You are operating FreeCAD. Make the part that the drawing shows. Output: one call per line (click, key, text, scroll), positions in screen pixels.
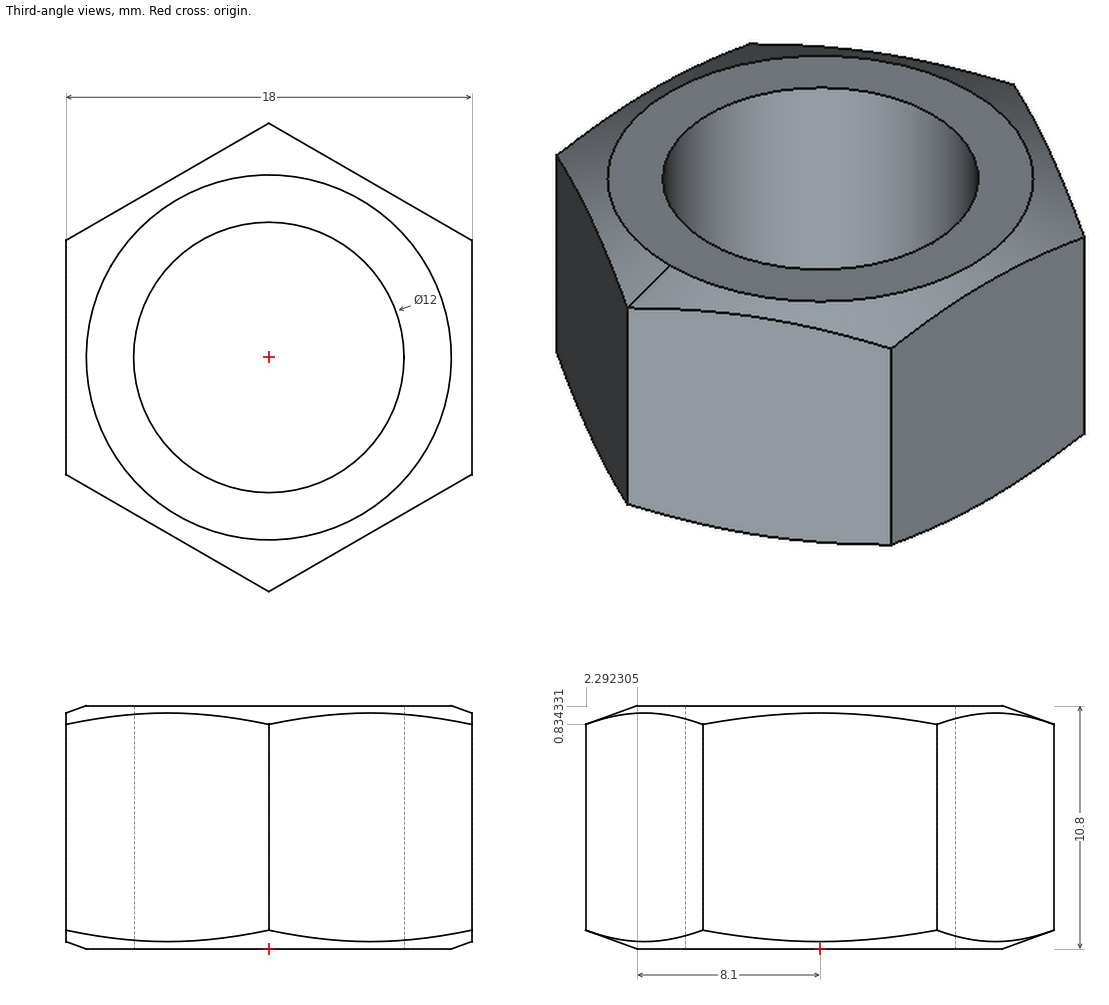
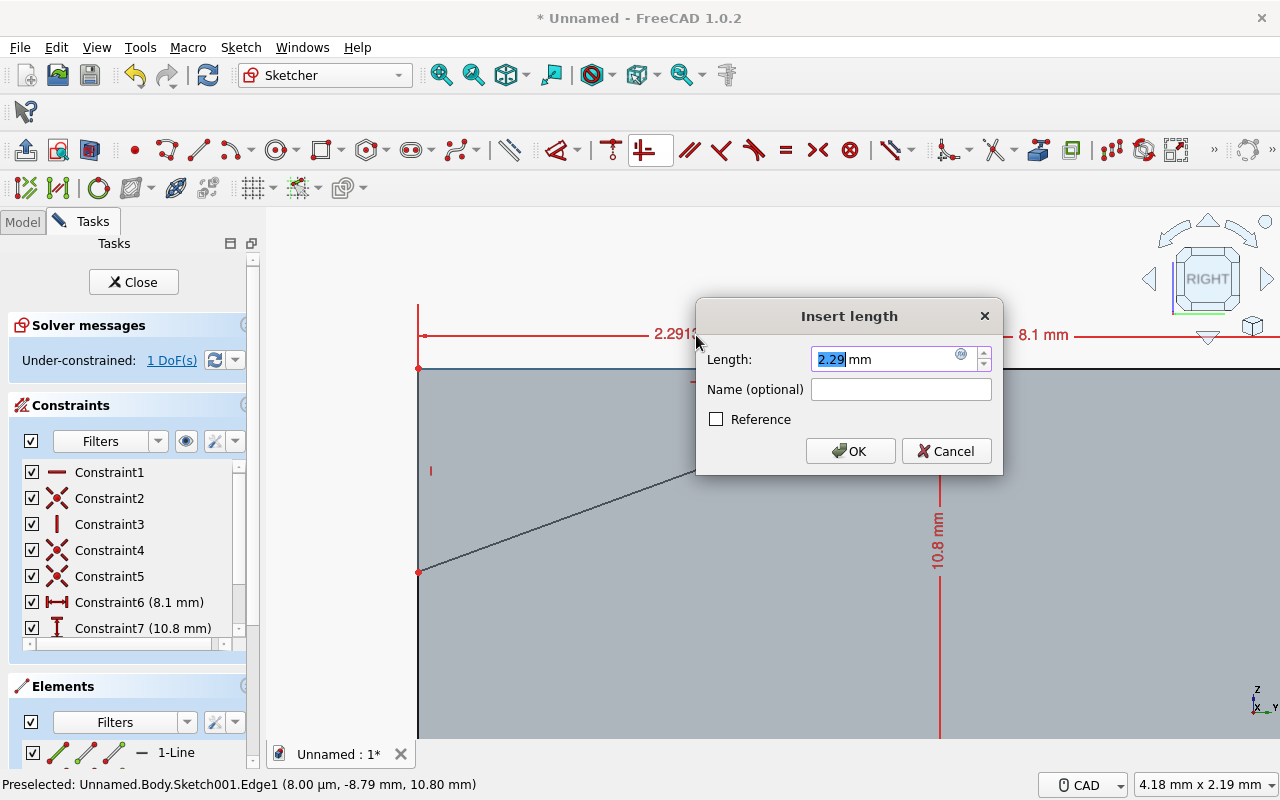
text(2.292305)
key(Return)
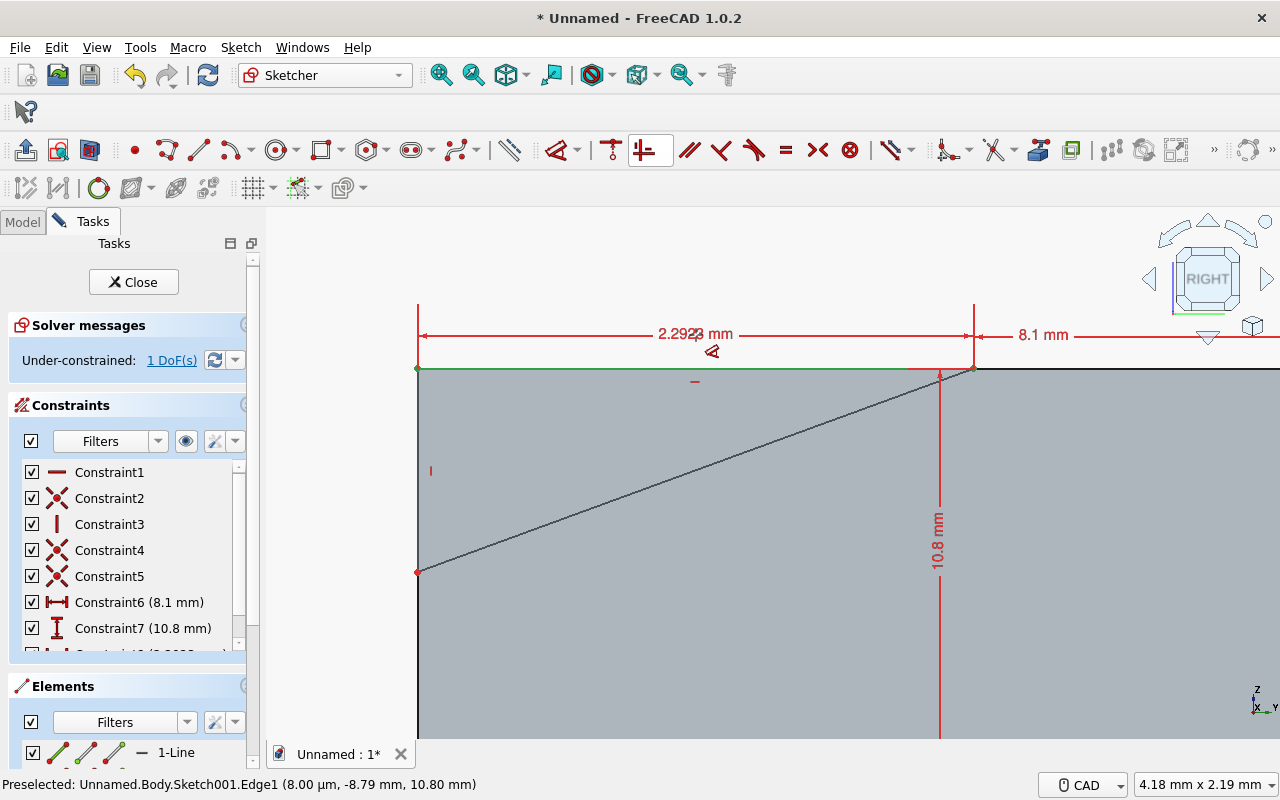
click(418, 430)
click(384, 470)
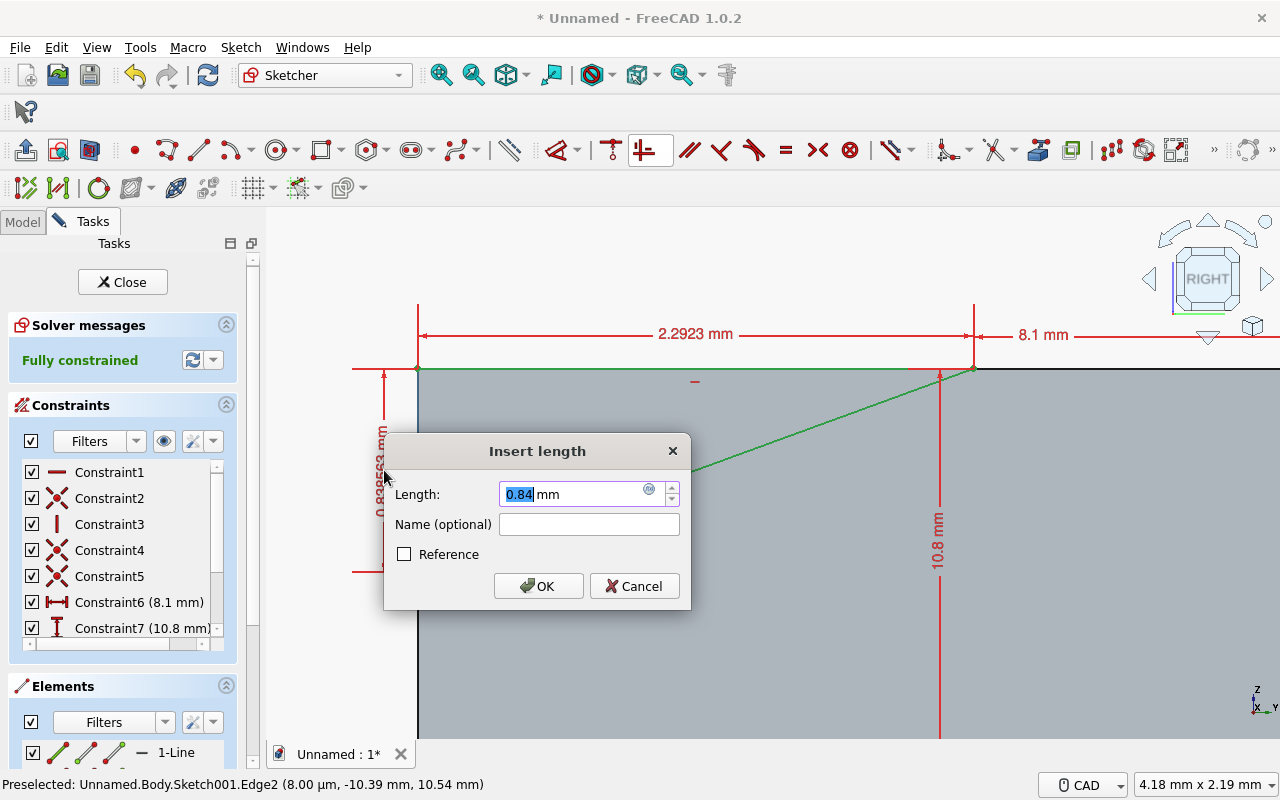
text(0.834331)
key(Return)
key(Escape)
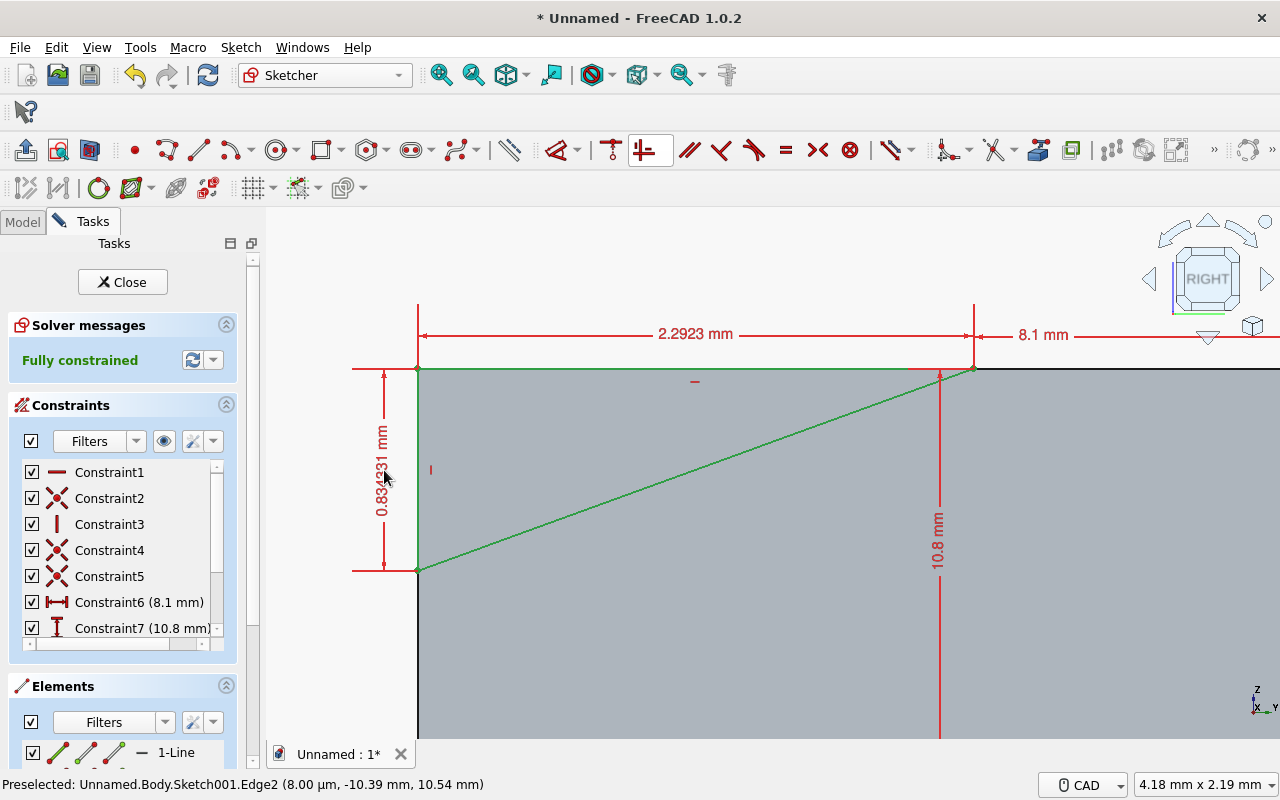
click(123, 282)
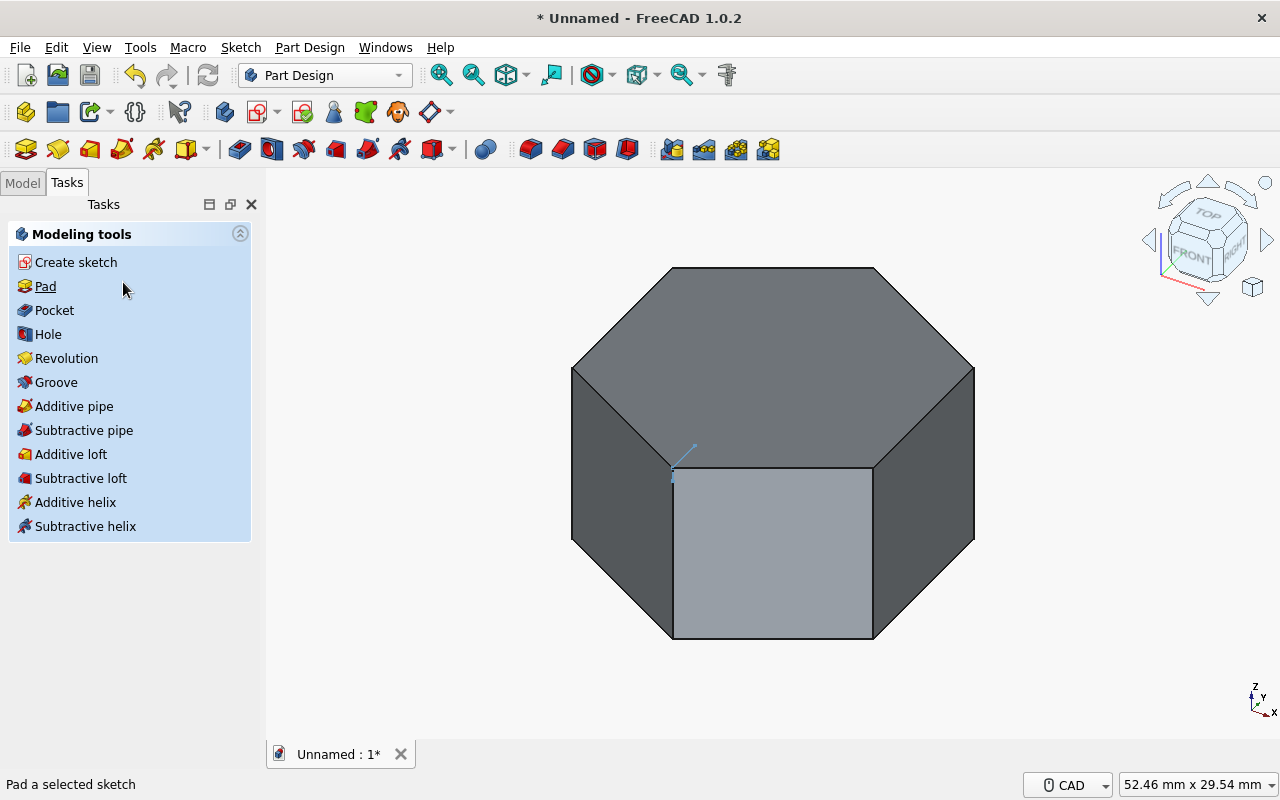
click(304, 150)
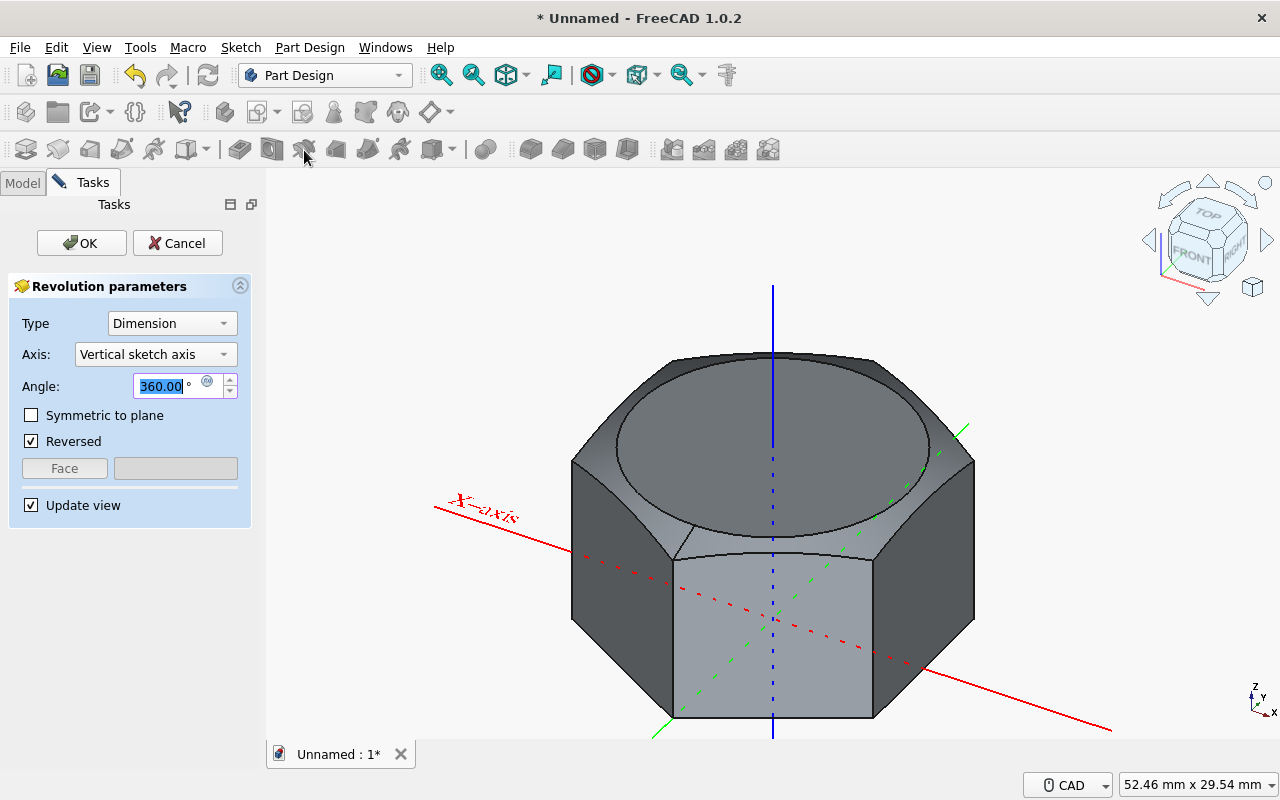
click(82, 243)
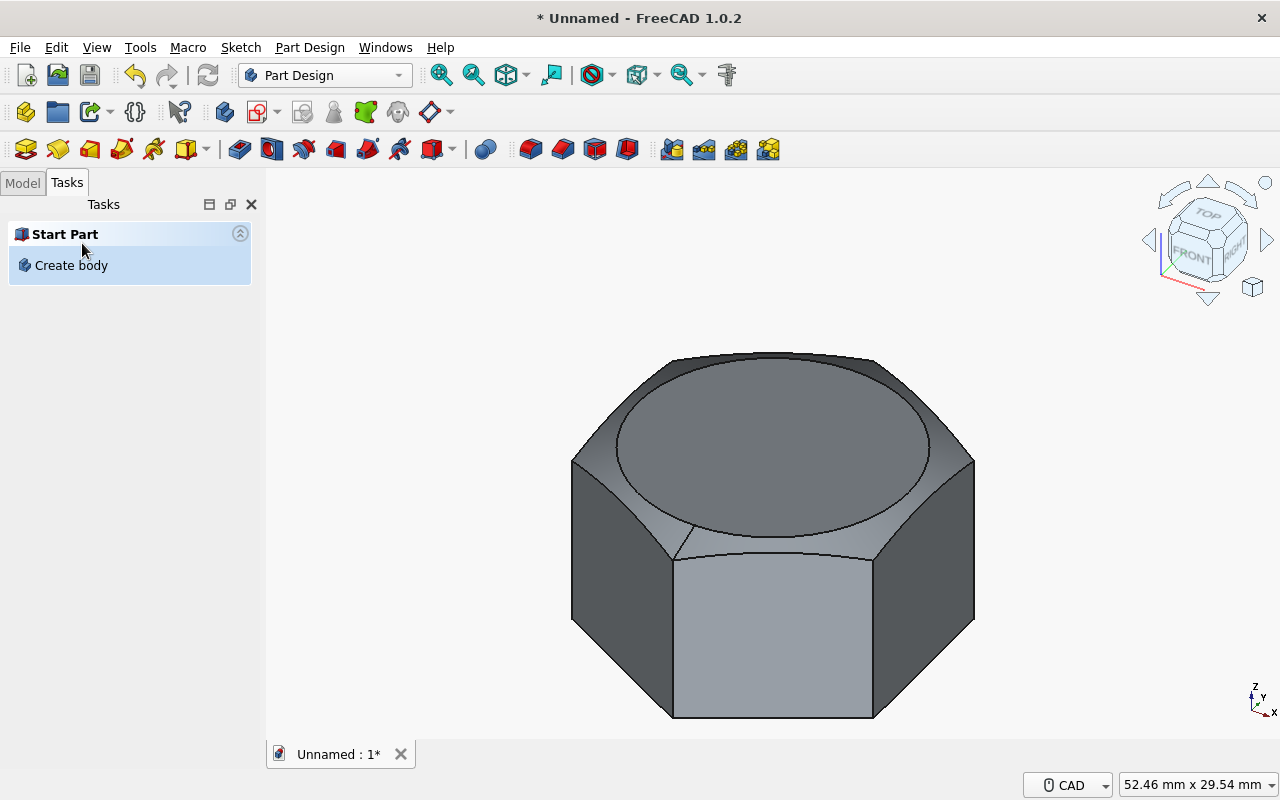
click(442, 76)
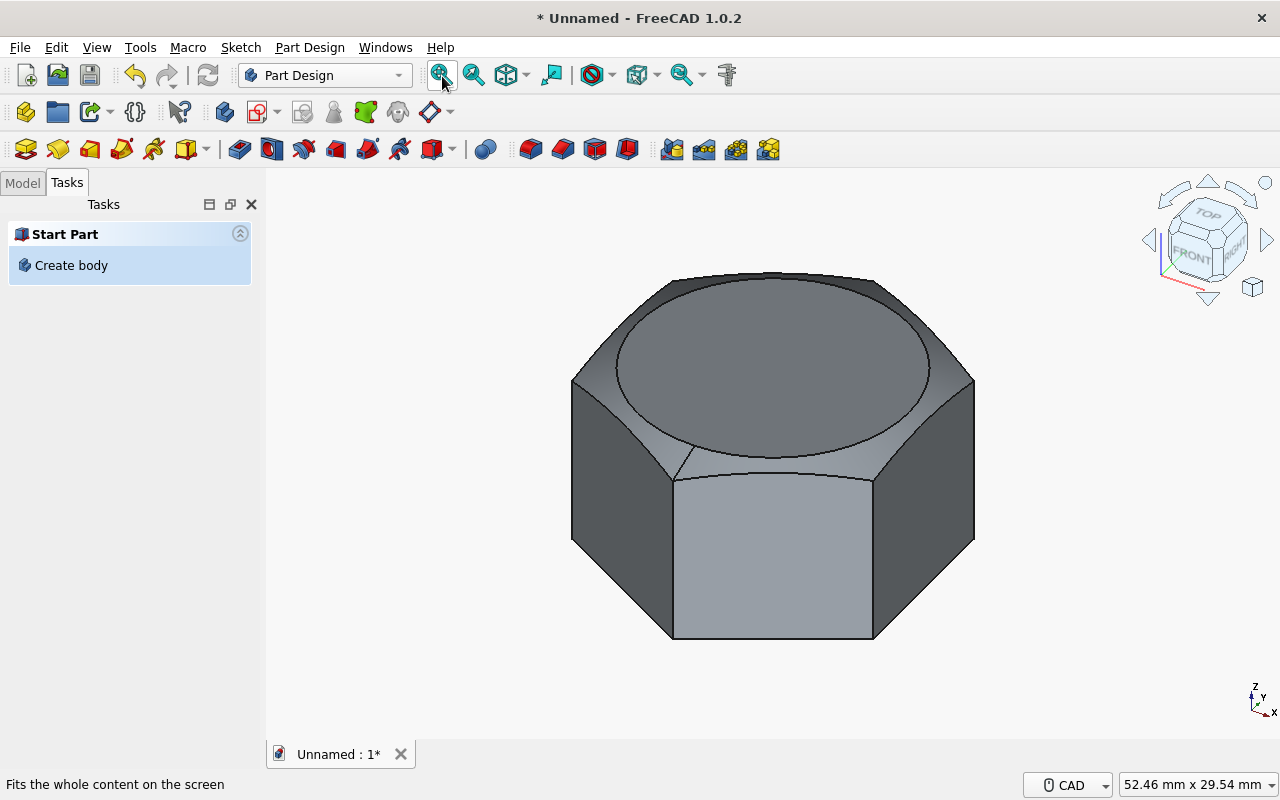
click(23, 182)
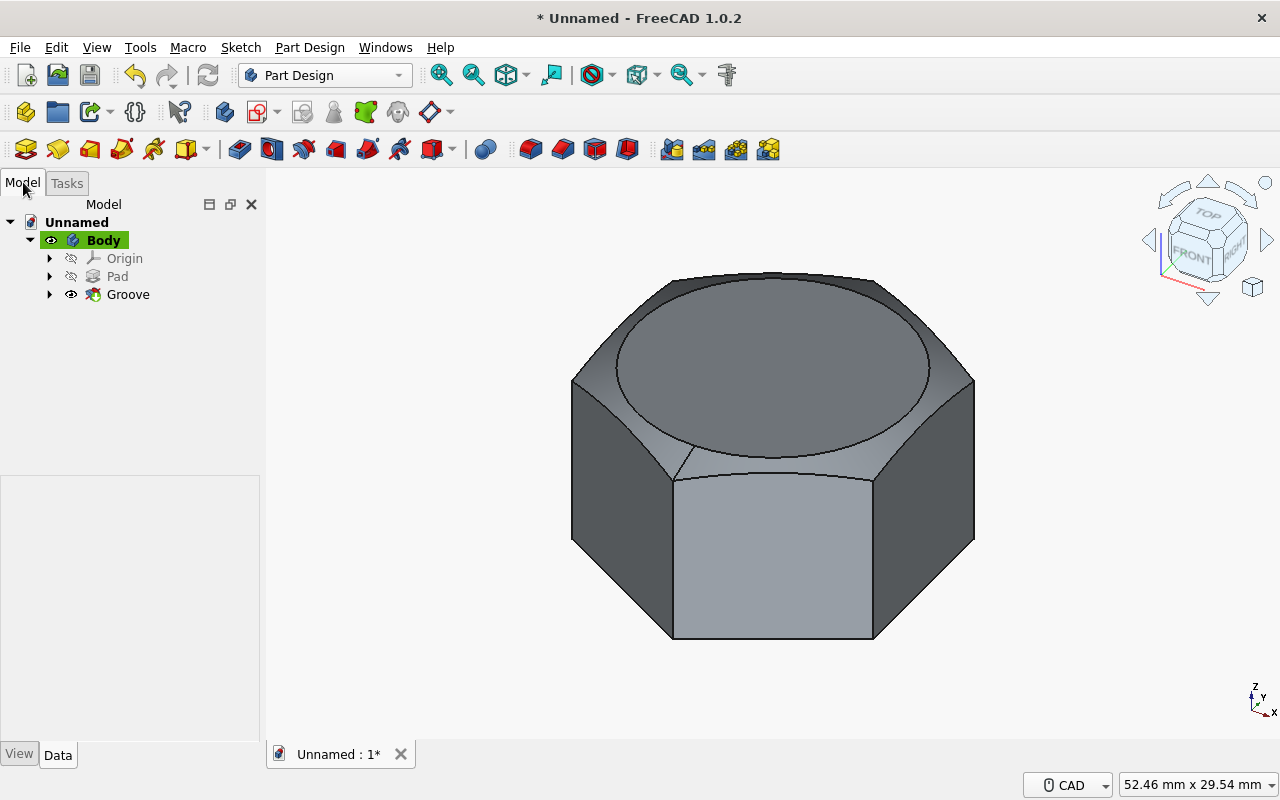
click(50, 258)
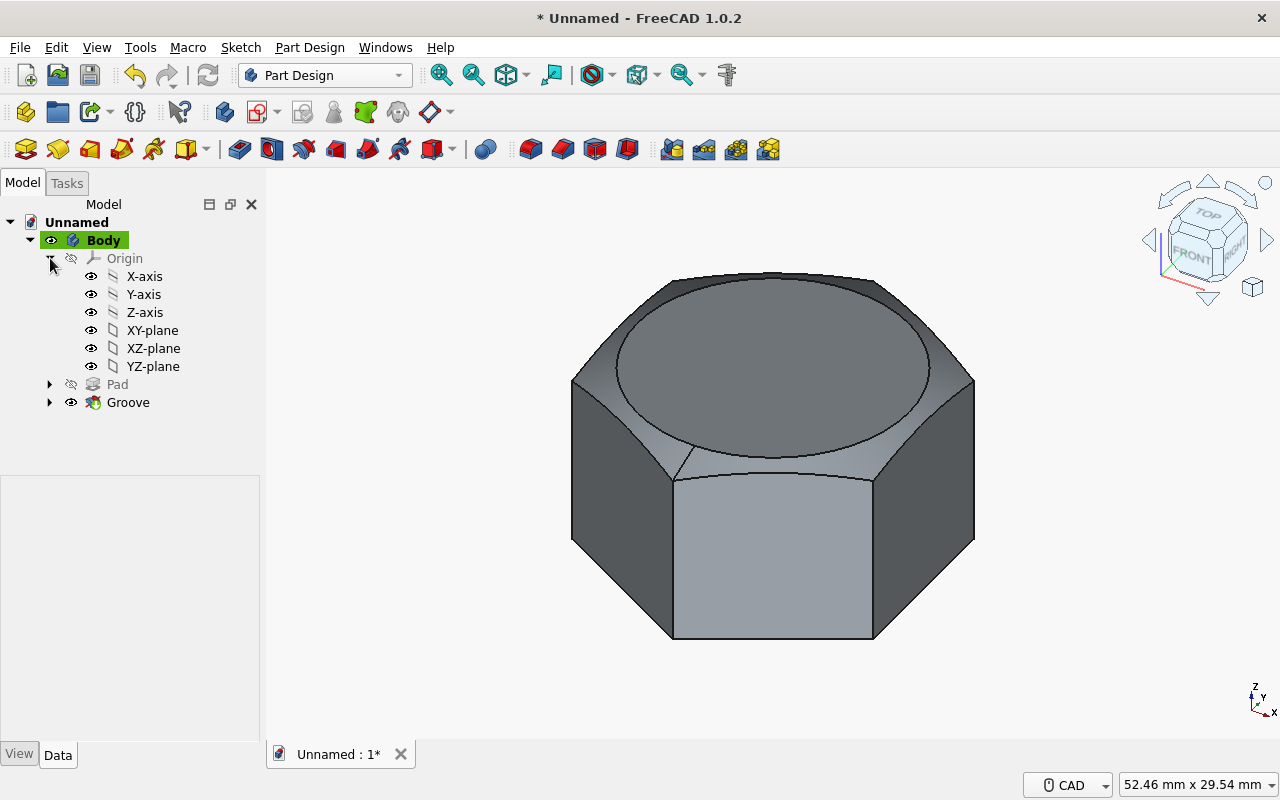
click(136, 330)